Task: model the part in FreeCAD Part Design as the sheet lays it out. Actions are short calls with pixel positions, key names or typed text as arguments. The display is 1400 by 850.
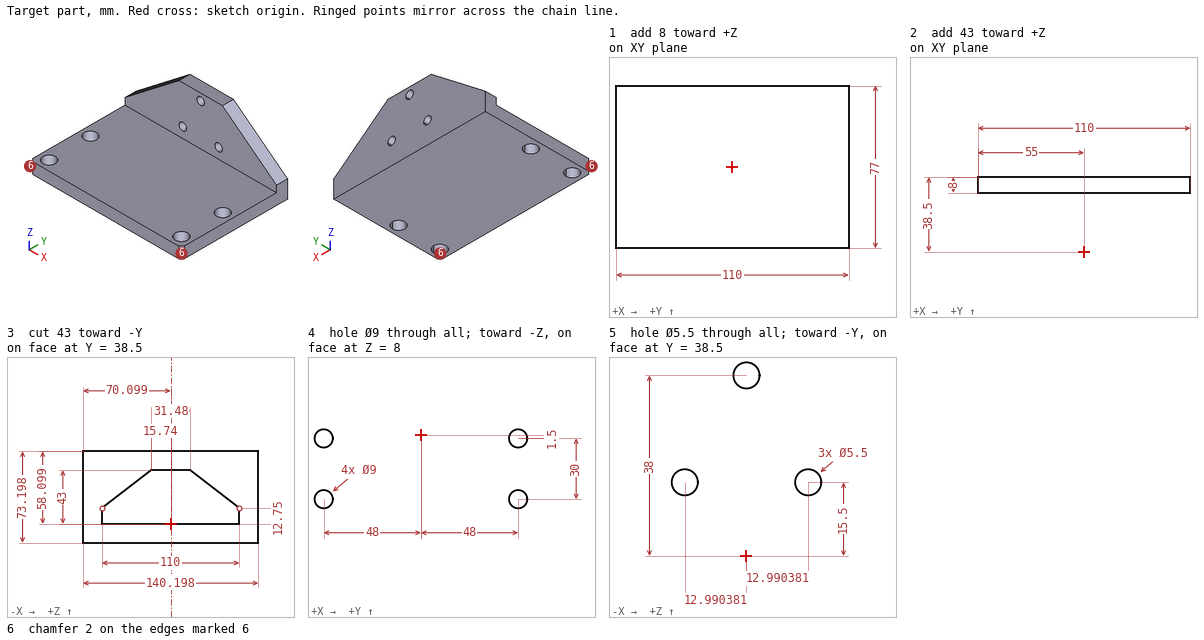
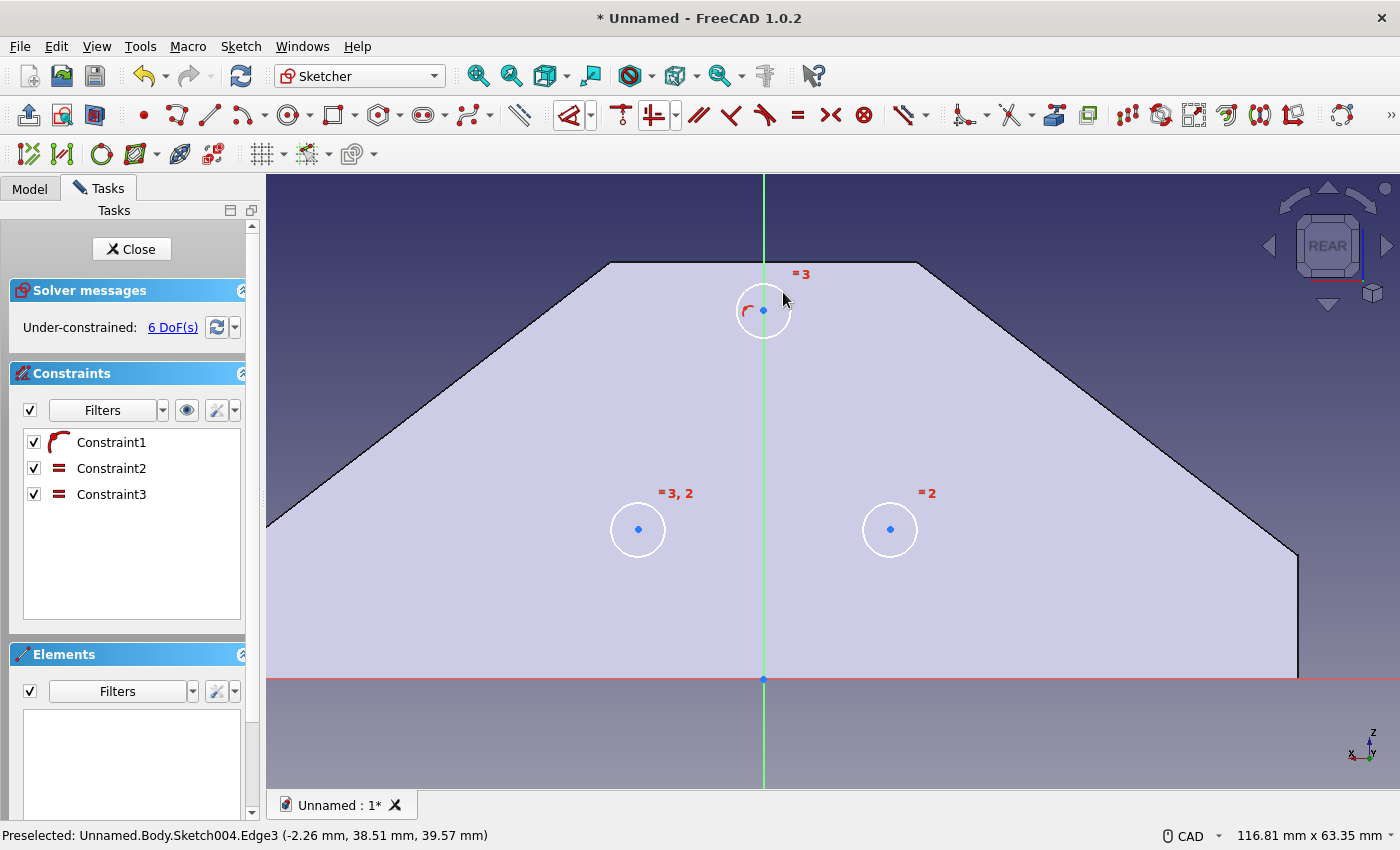
click(890, 530)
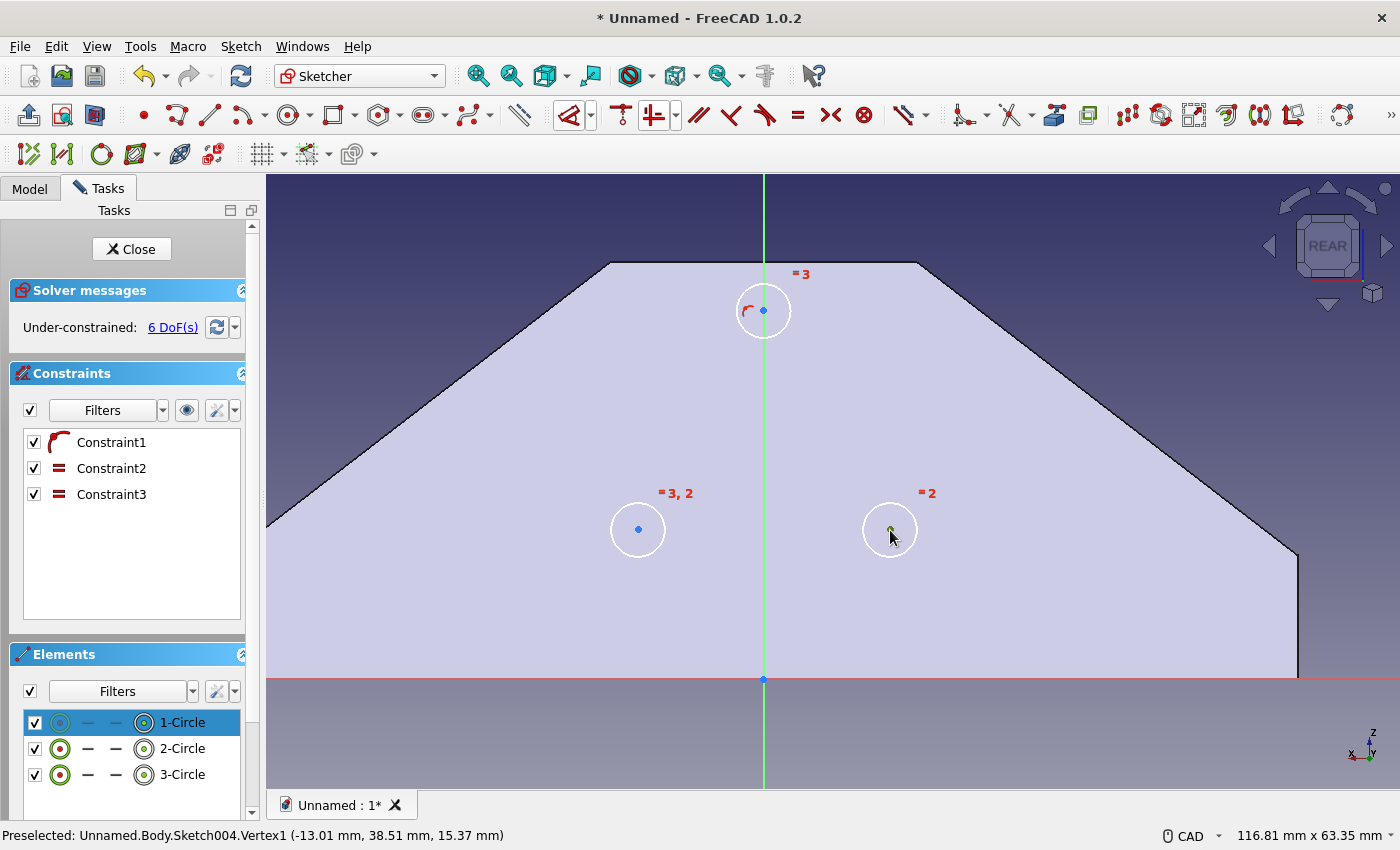
click(638, 530)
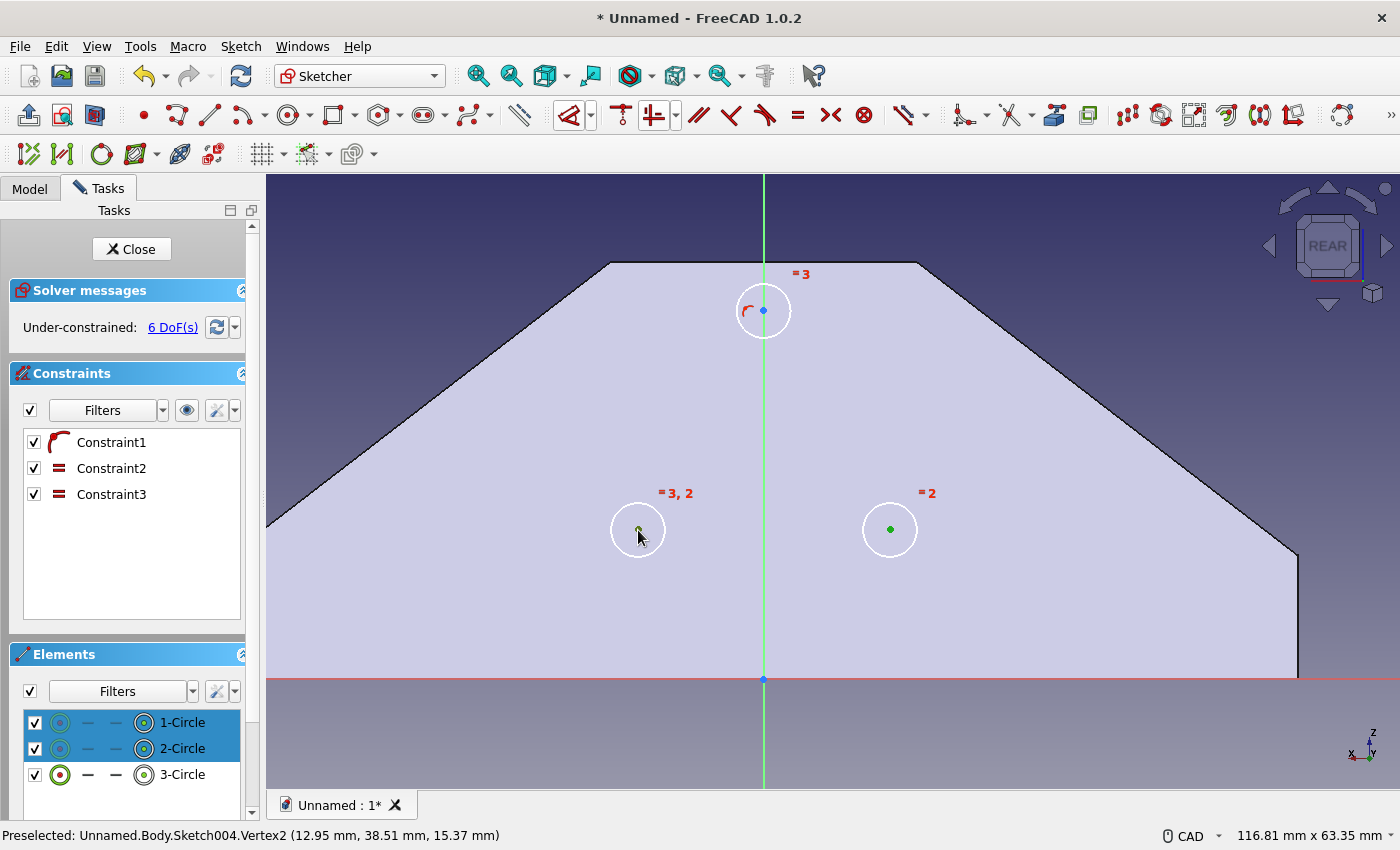
key(h)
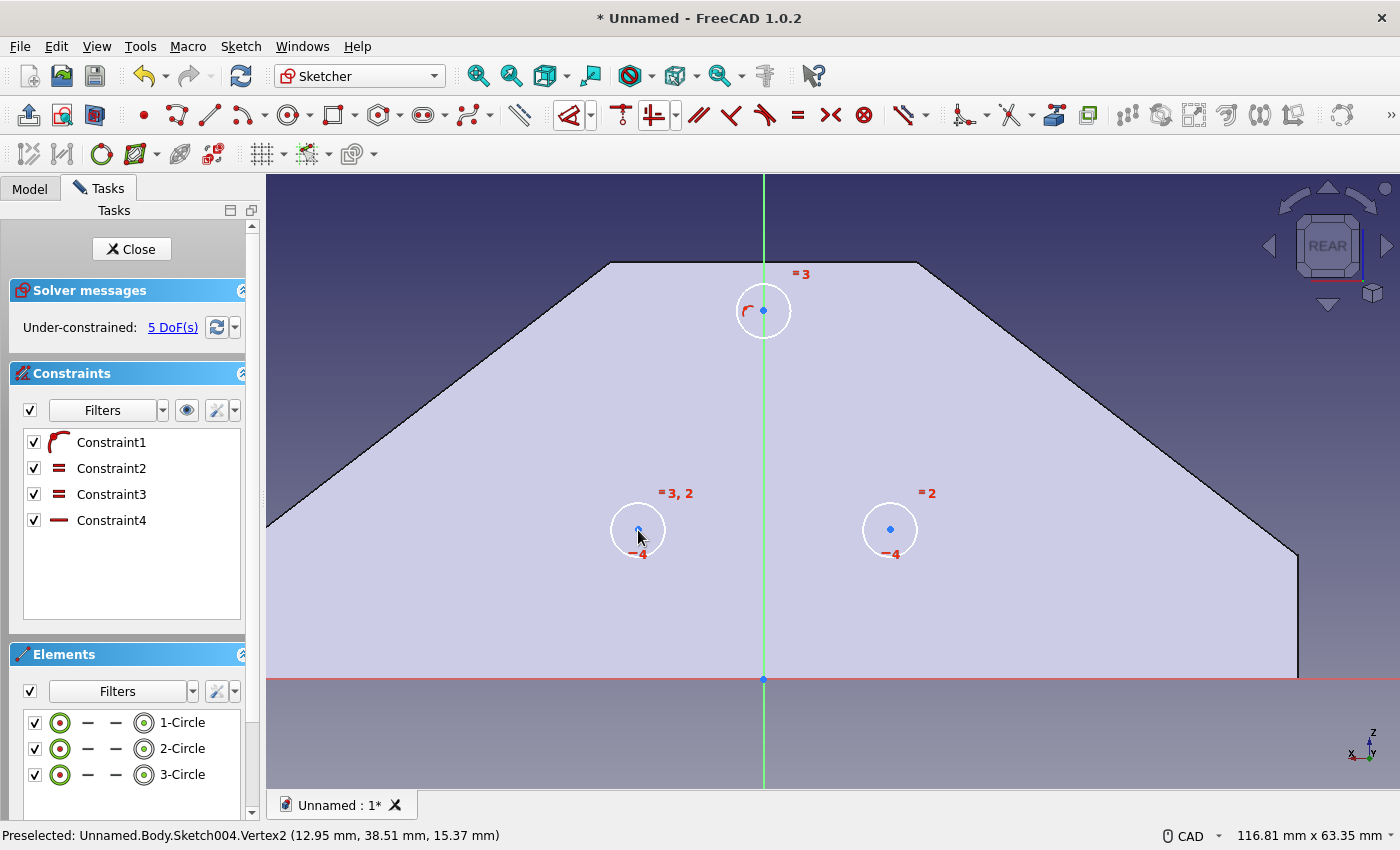
click(909, 511)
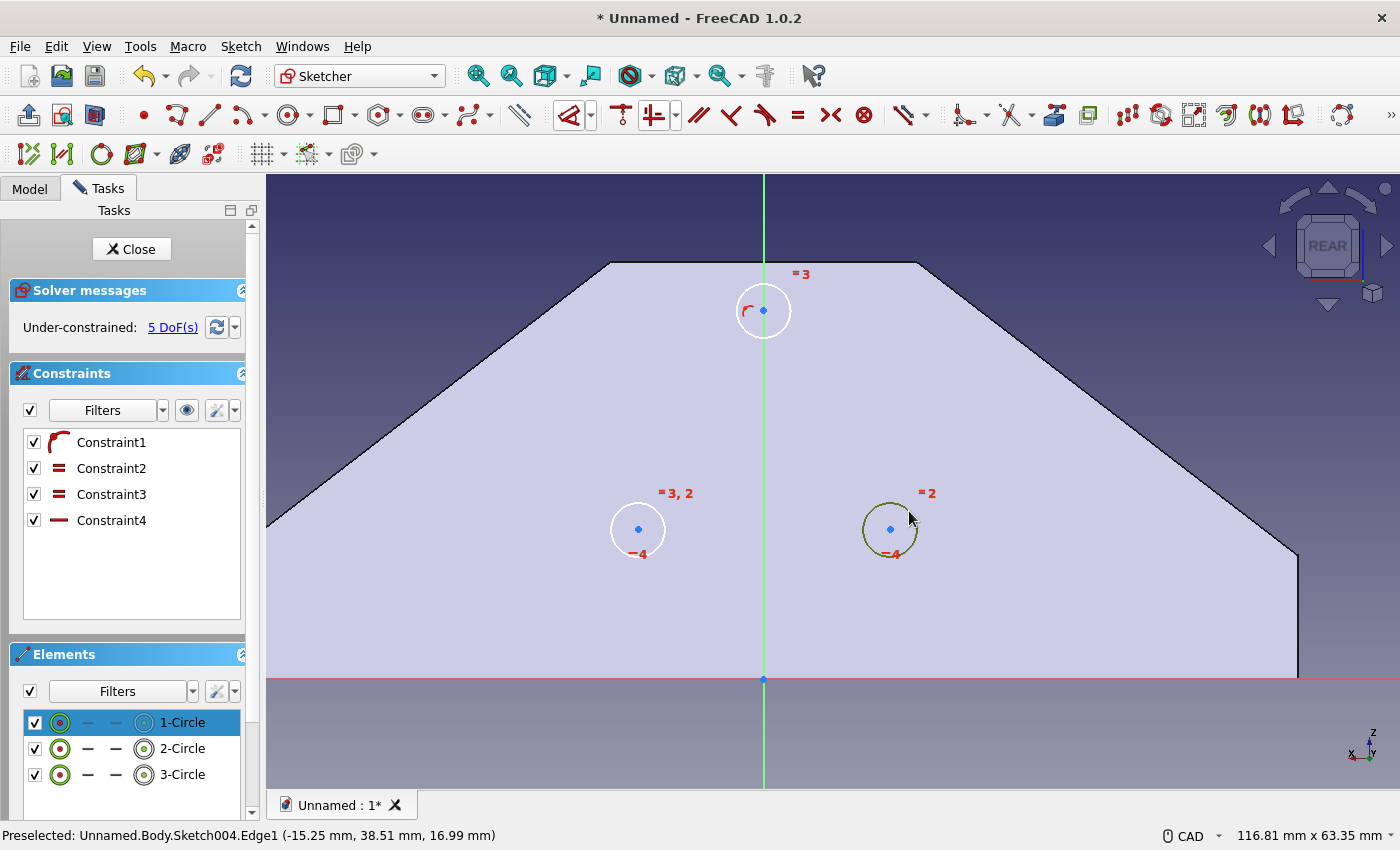
click(590, 116)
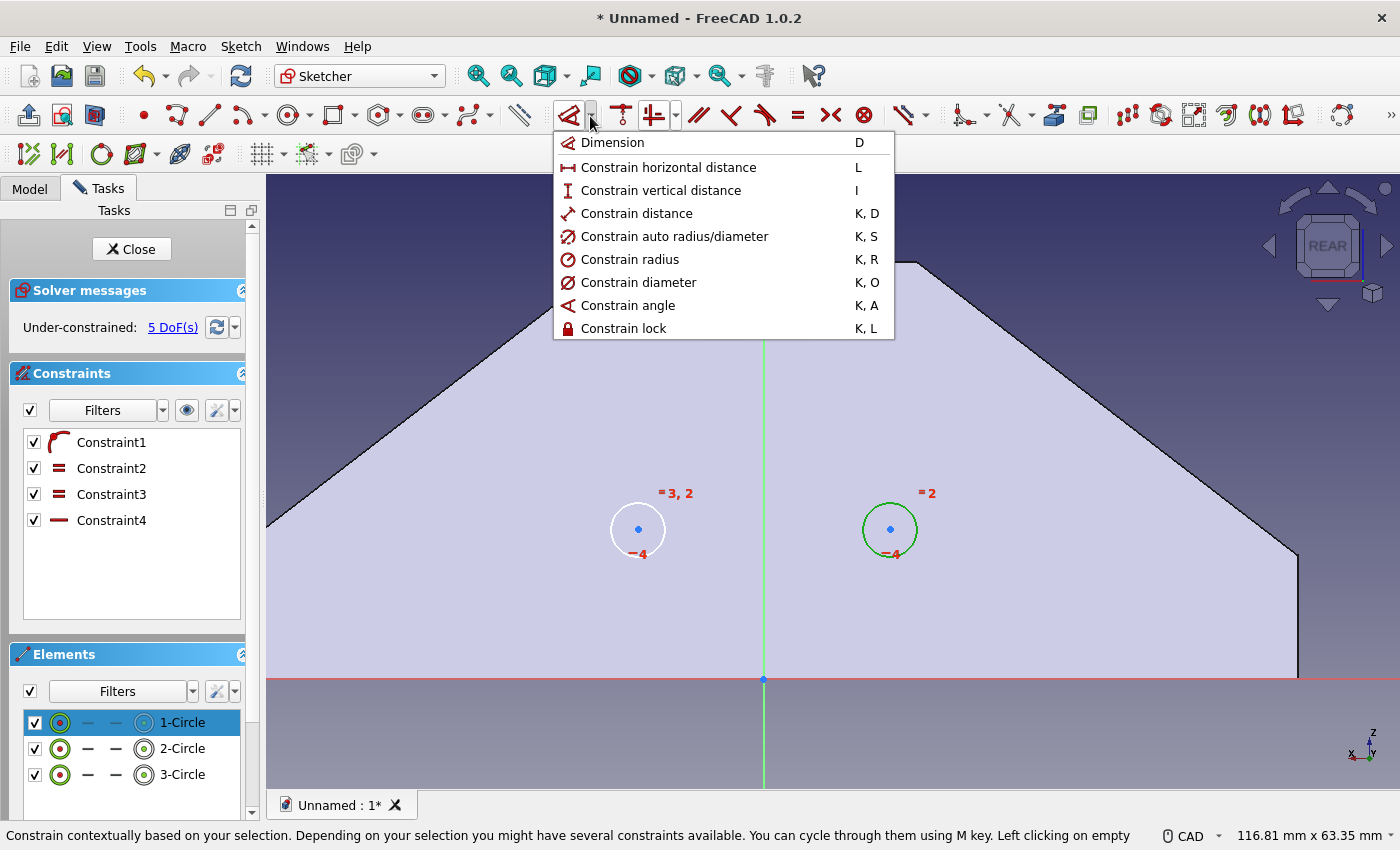
click(724, 282)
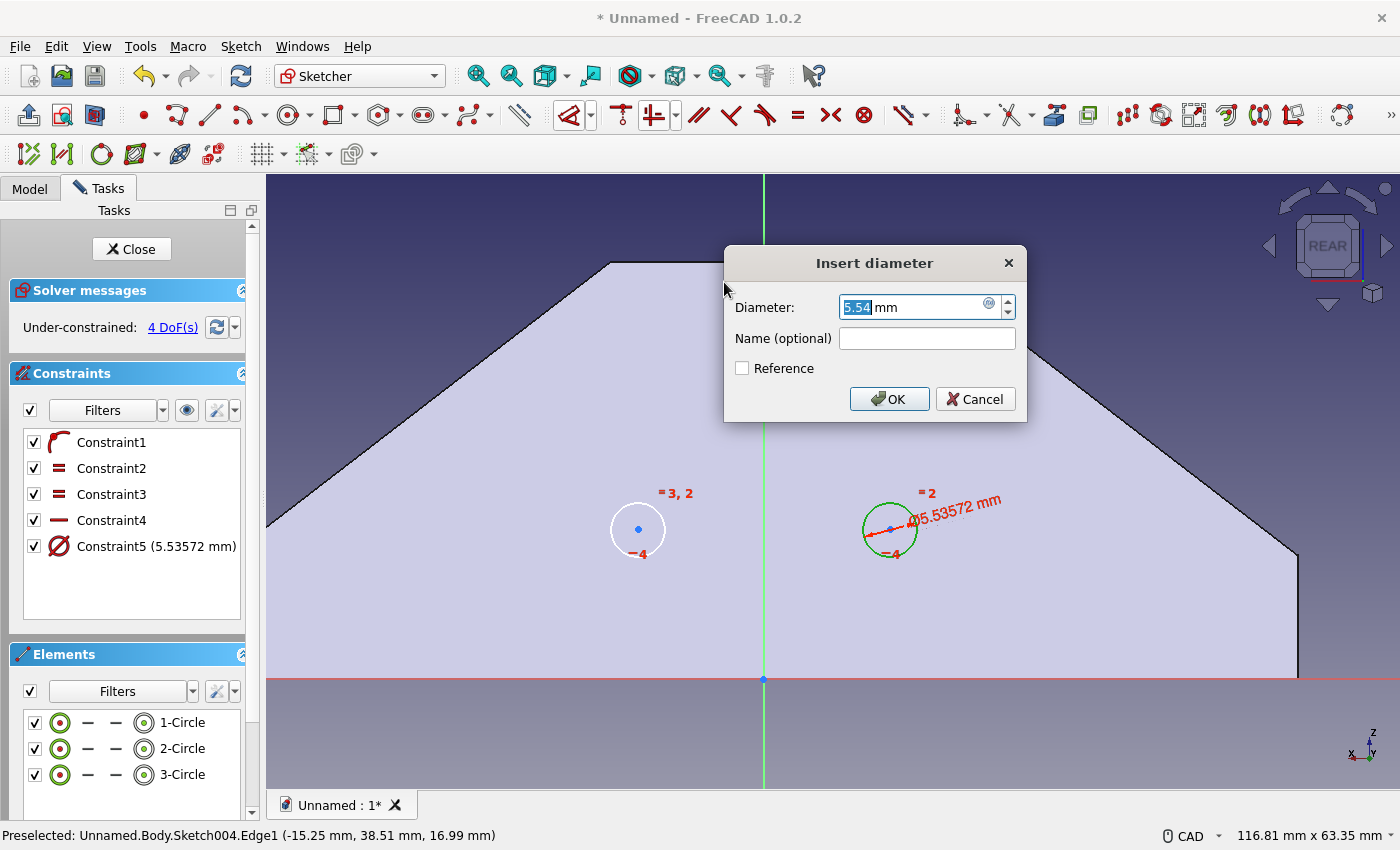
text(5.5)
key(Return)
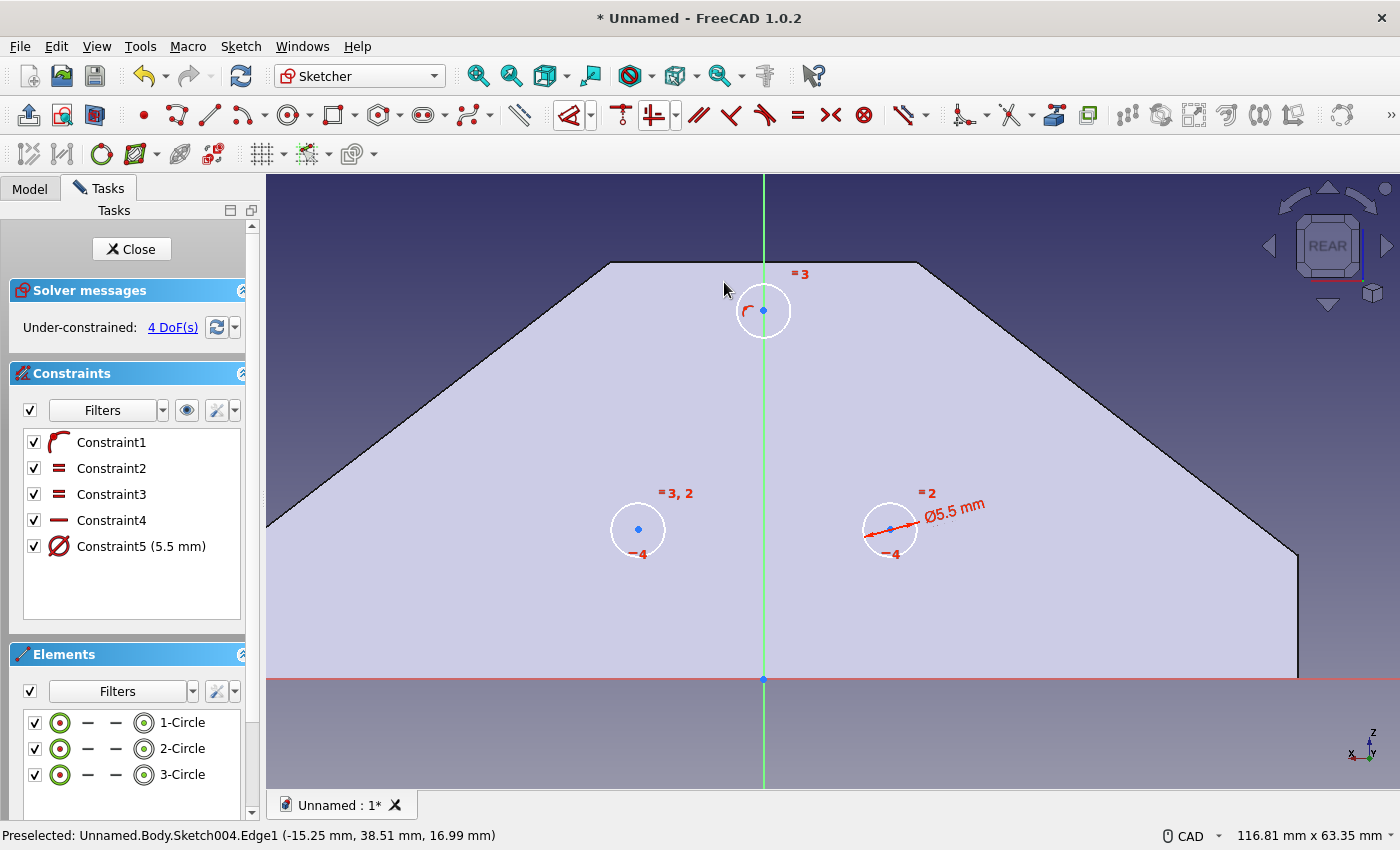
click(764, 311)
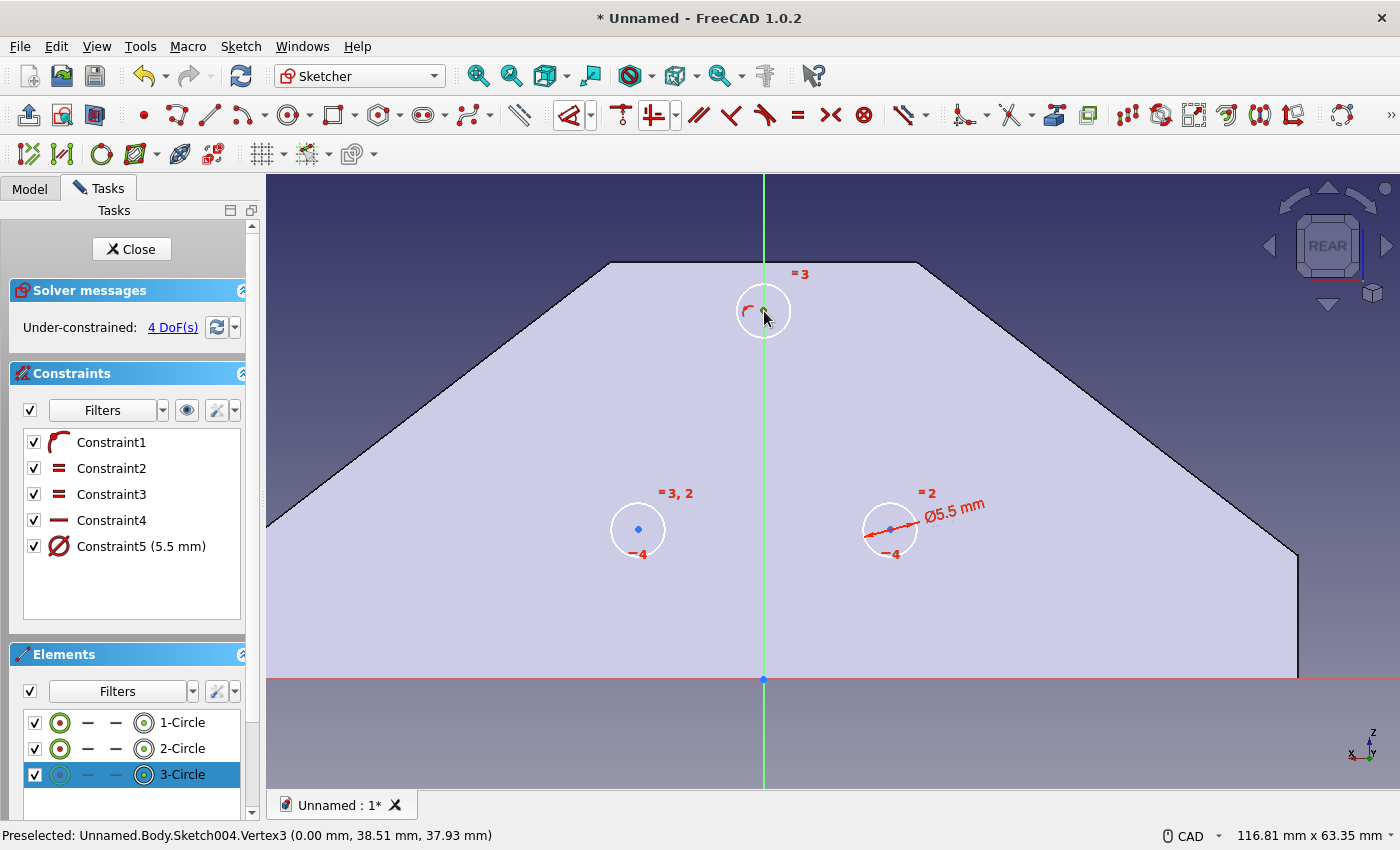
key(i)